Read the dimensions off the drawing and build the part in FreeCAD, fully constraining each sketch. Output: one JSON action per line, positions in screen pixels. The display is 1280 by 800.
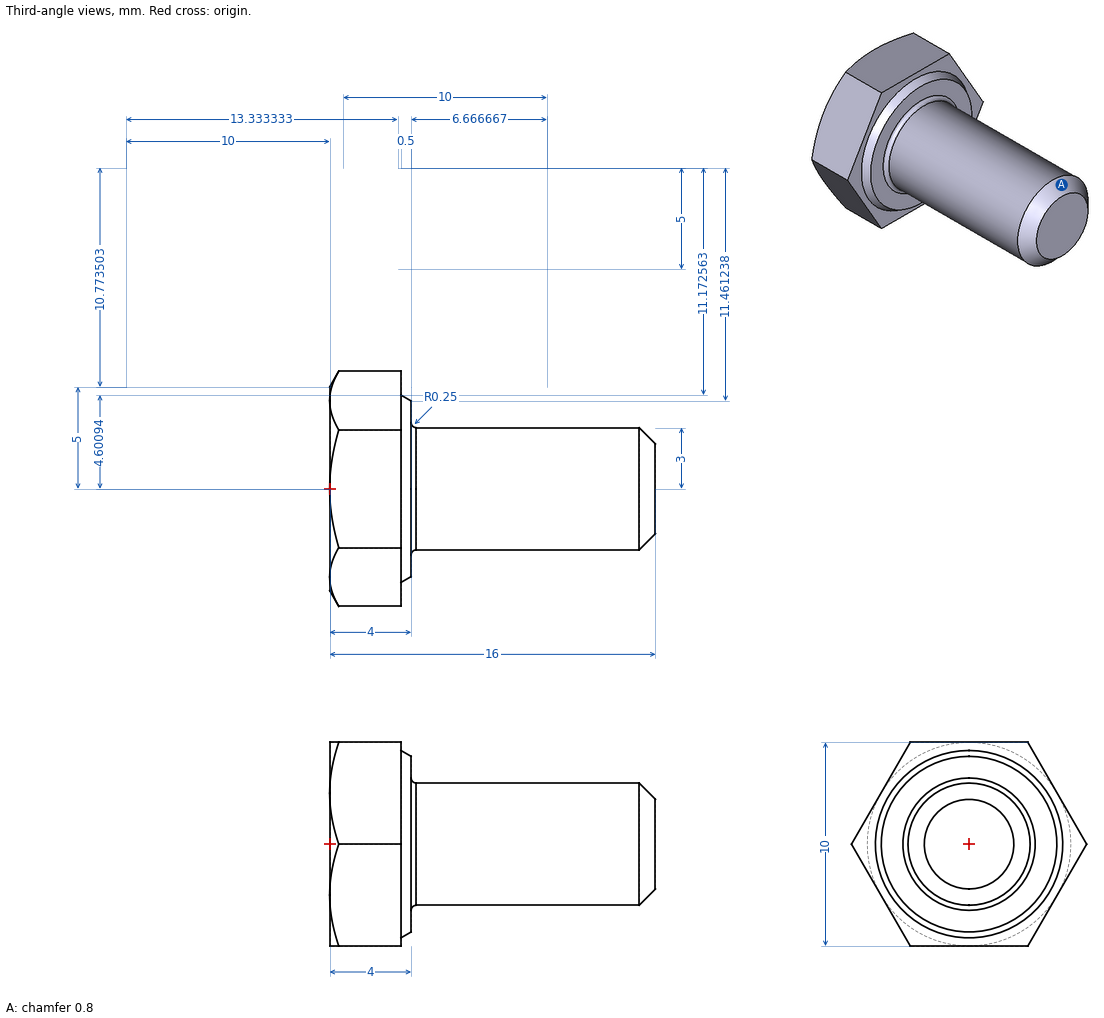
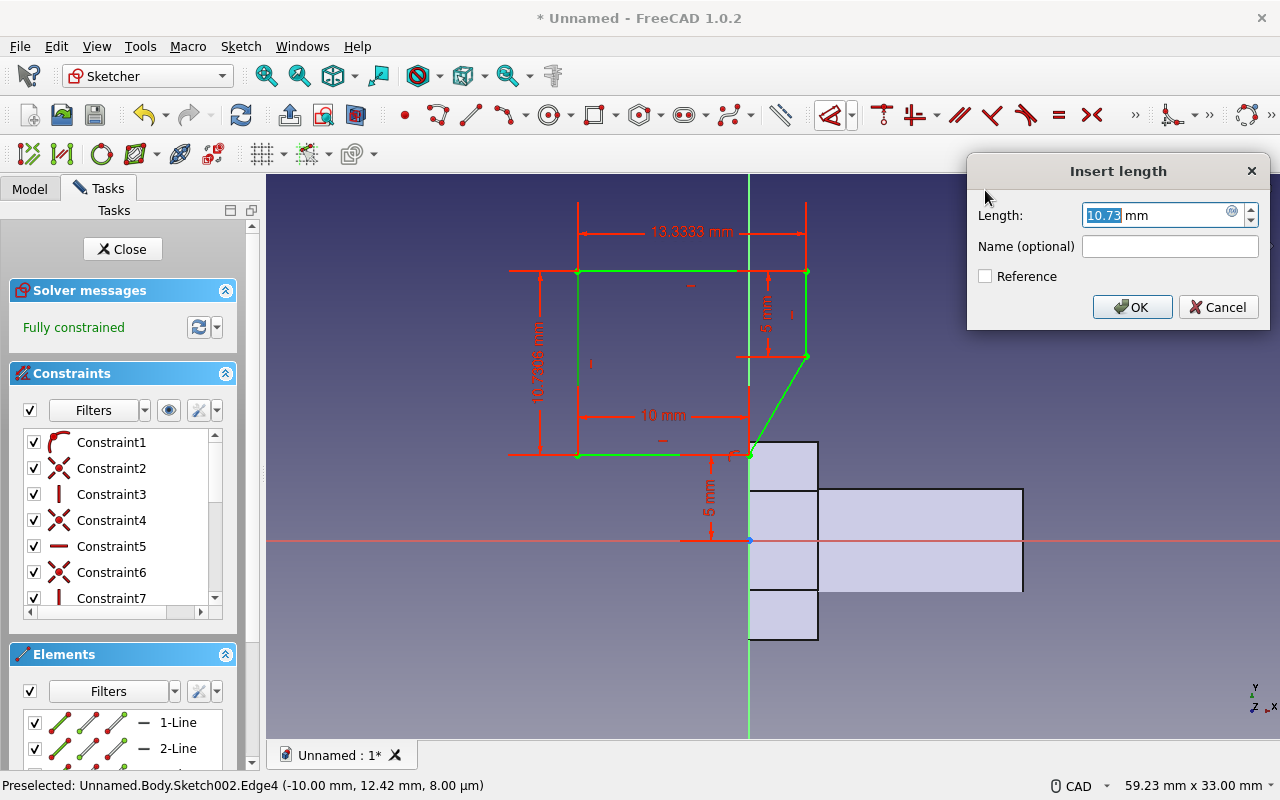
{"action": "type", "text": "10.773503"}
{"action": "key", "text": "Return"}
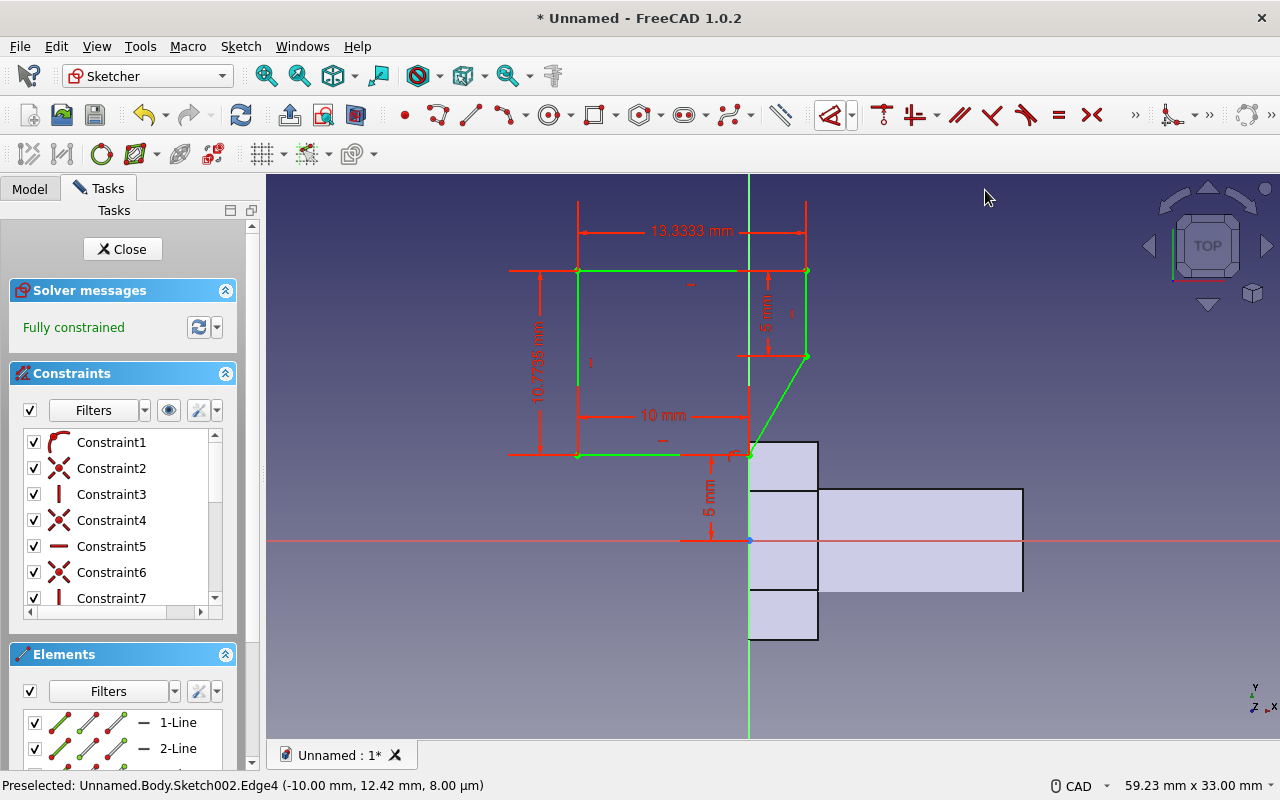
{"action": "left_click", "coordinate": [123, 249]}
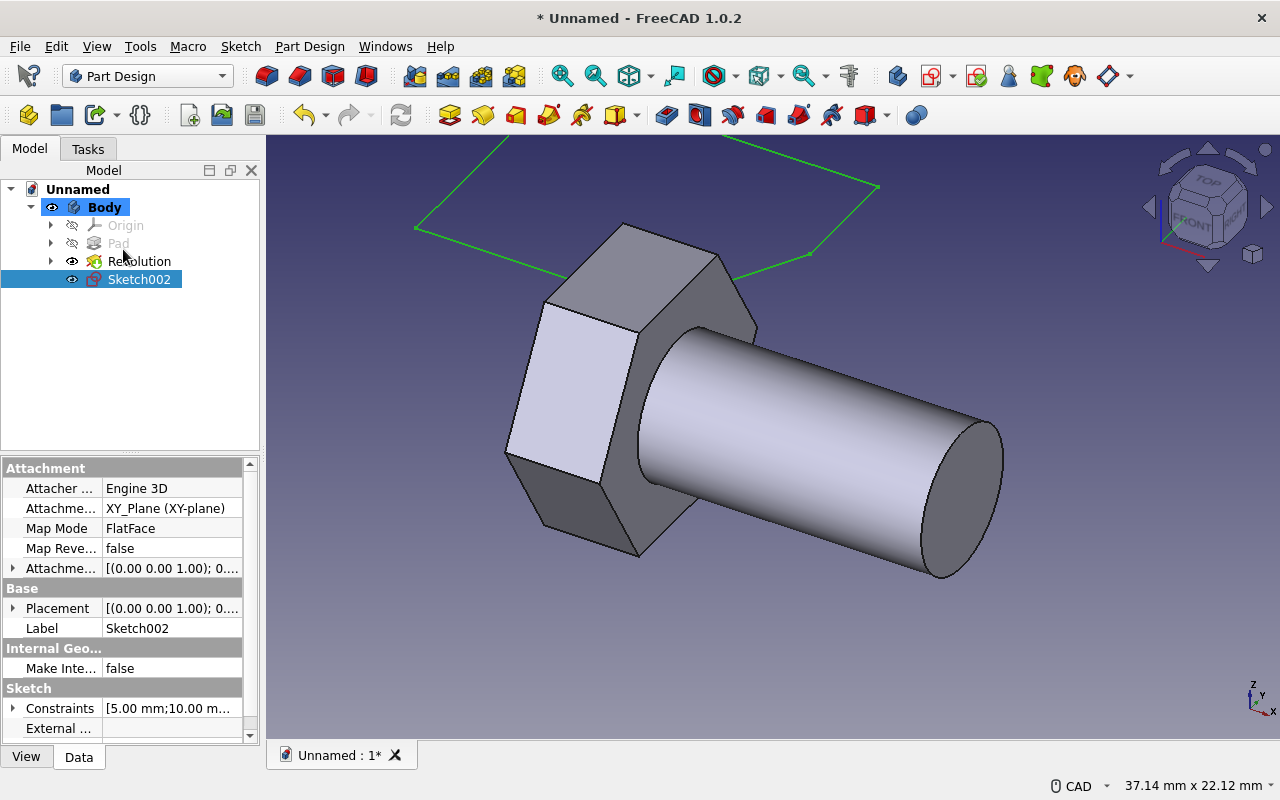
{"action": "left_click", "coordinate": [733, 116]}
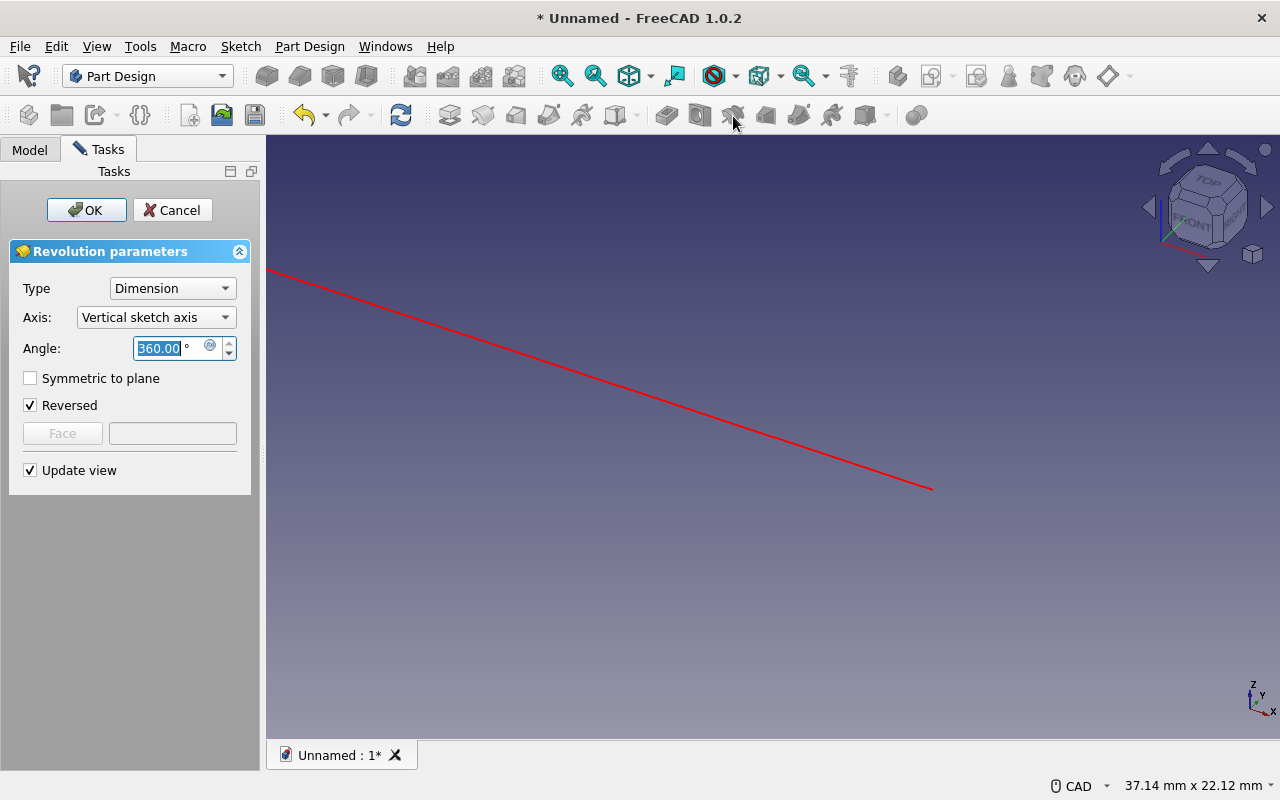
{"action": "left_click", "coordinate": [157, 318]}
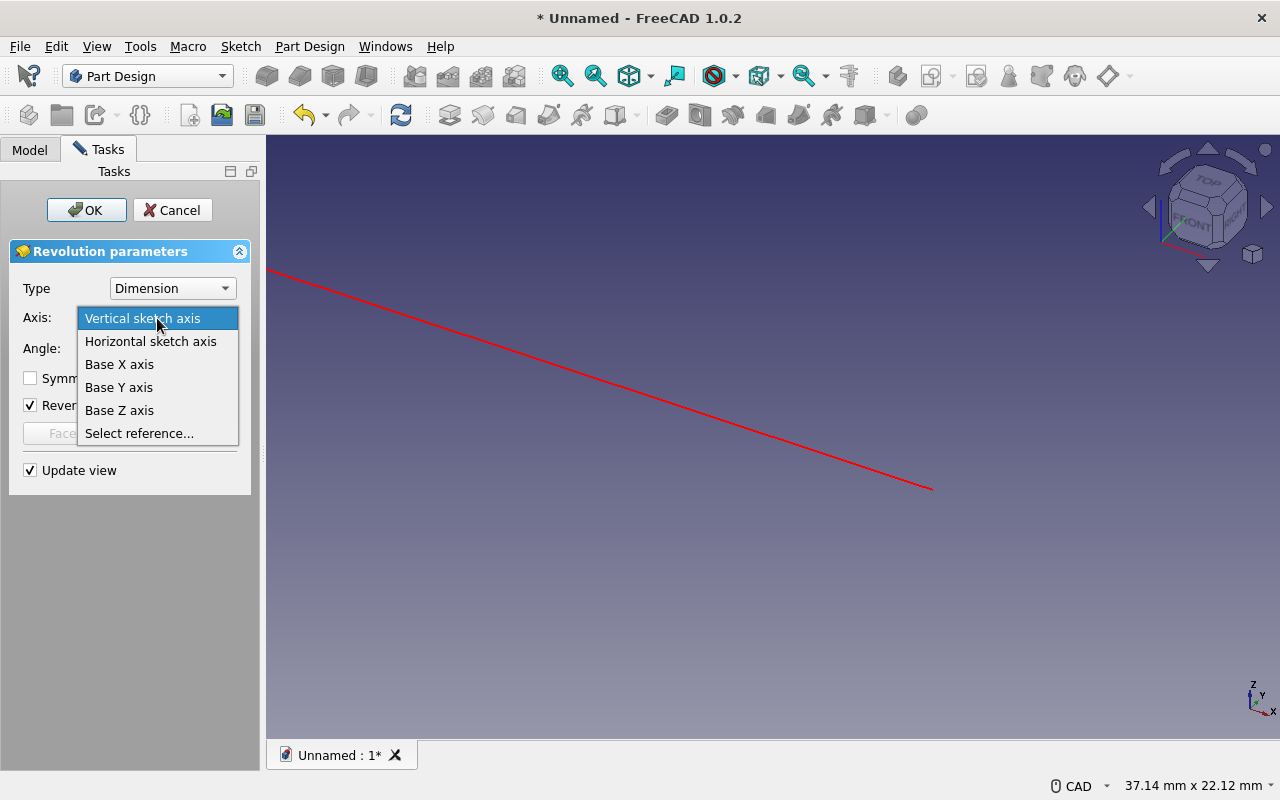
{"action": "left_click", "coordinate": [156, 342]}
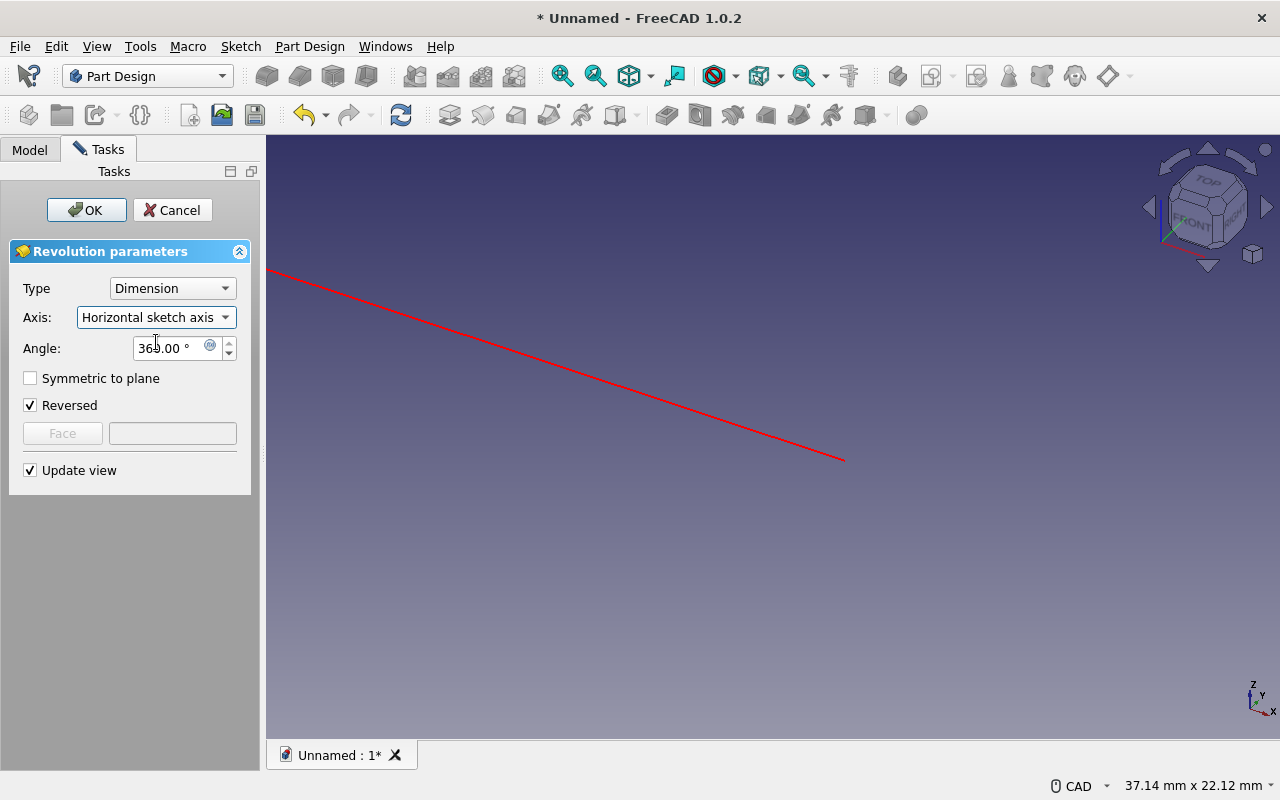
{"action": "left_click", "coordinate": [87, 210]}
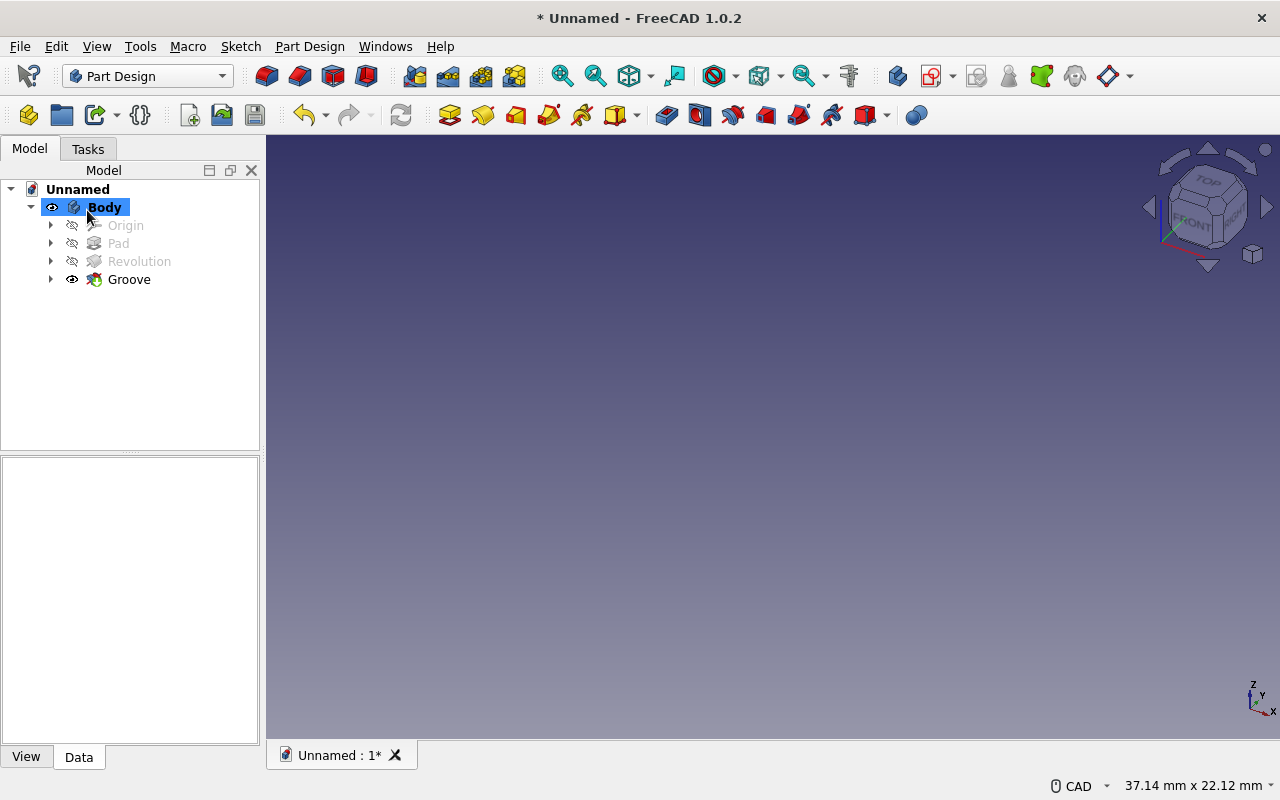
{"action": "left_click", "coordinate": [563, 76]}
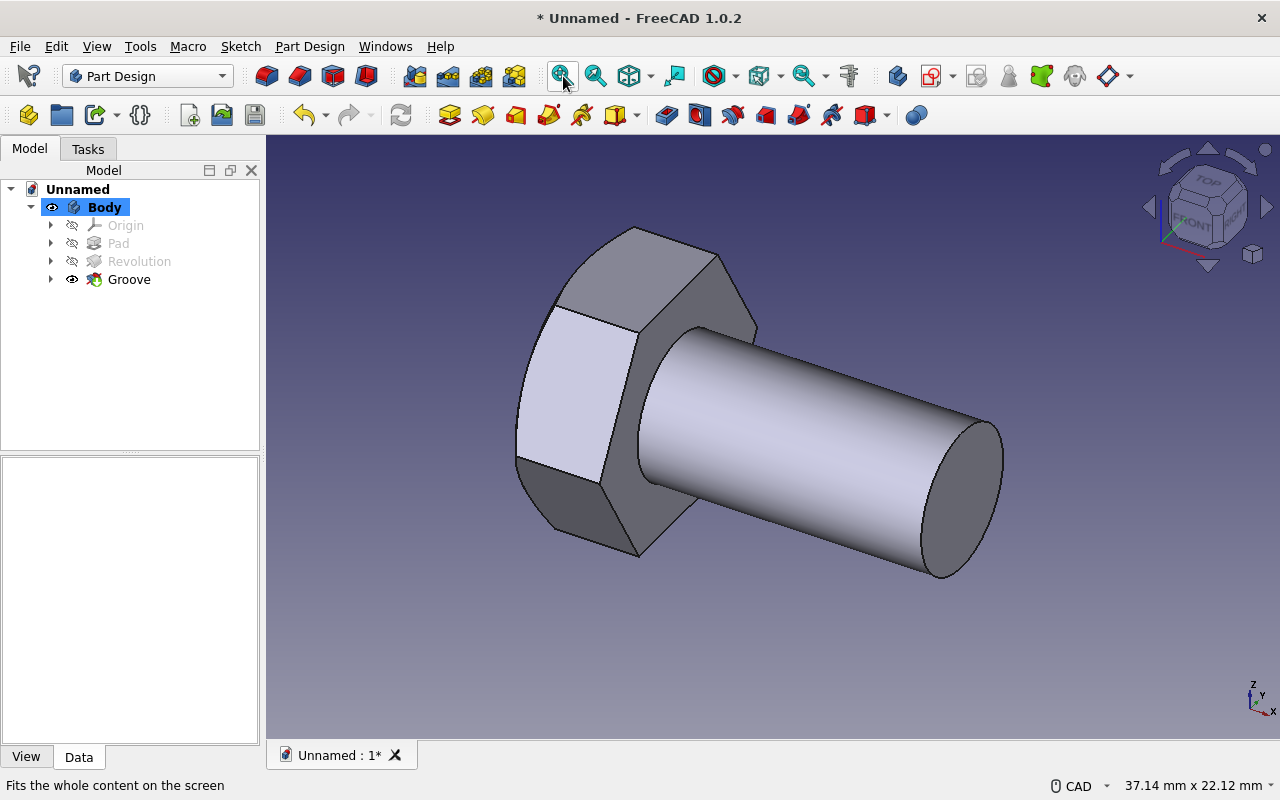
{"action": "left_click", "coordinate": [930, 76]}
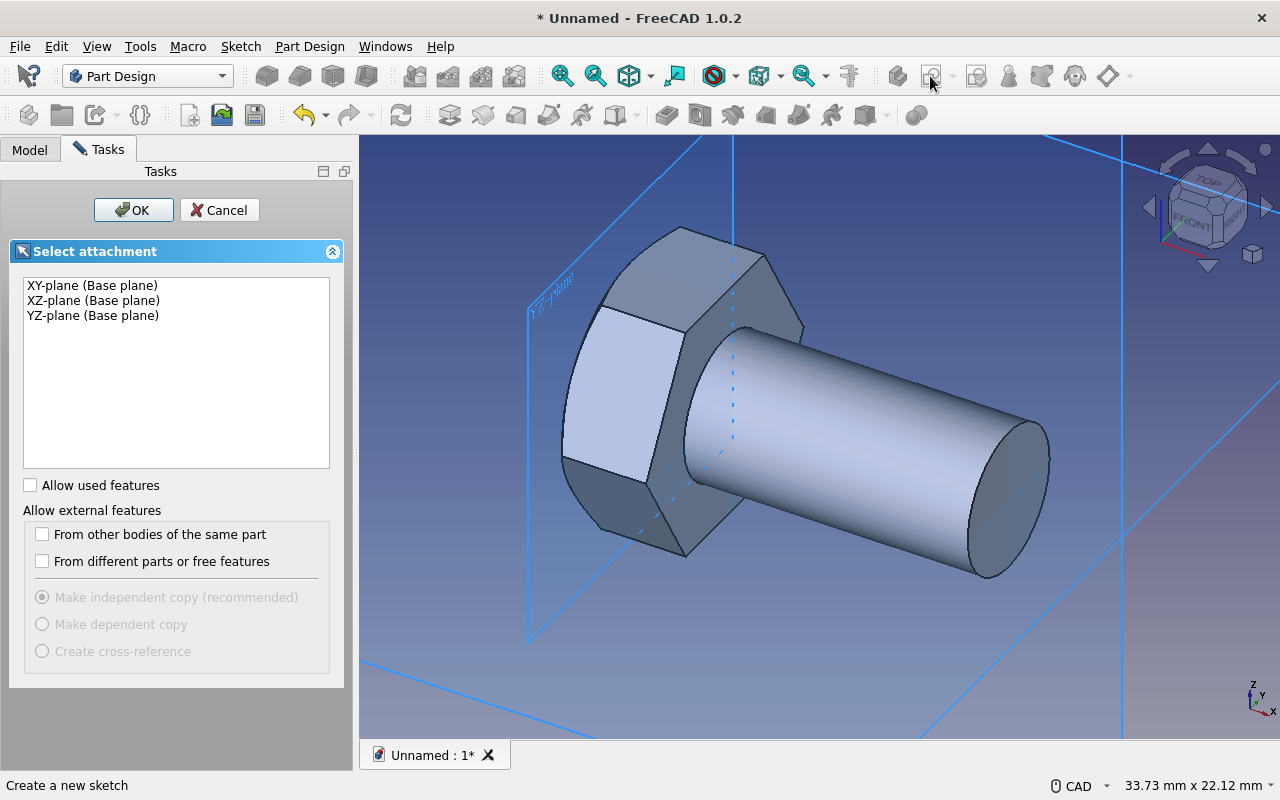
{"action": "left_click", "coordinate": [84, 286]}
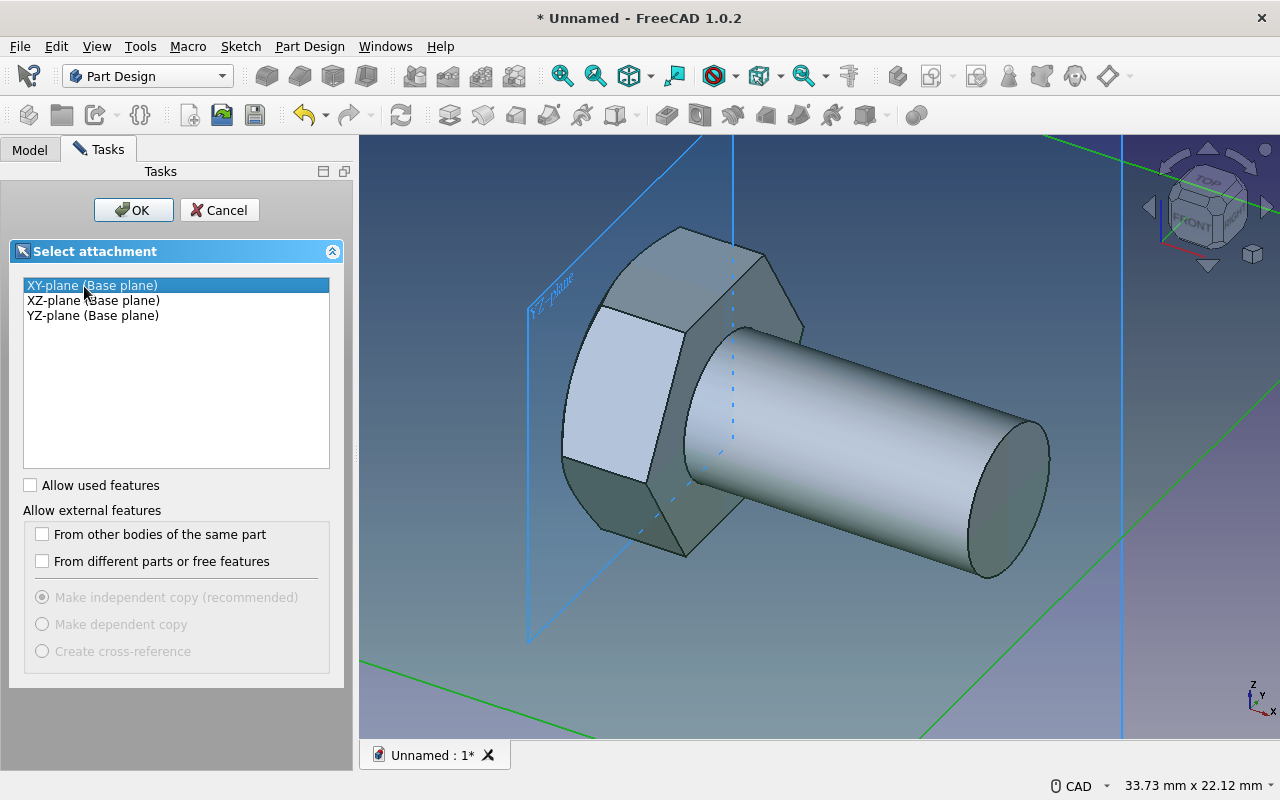
{"action": "left_click", "coordinate": [134, 210]}